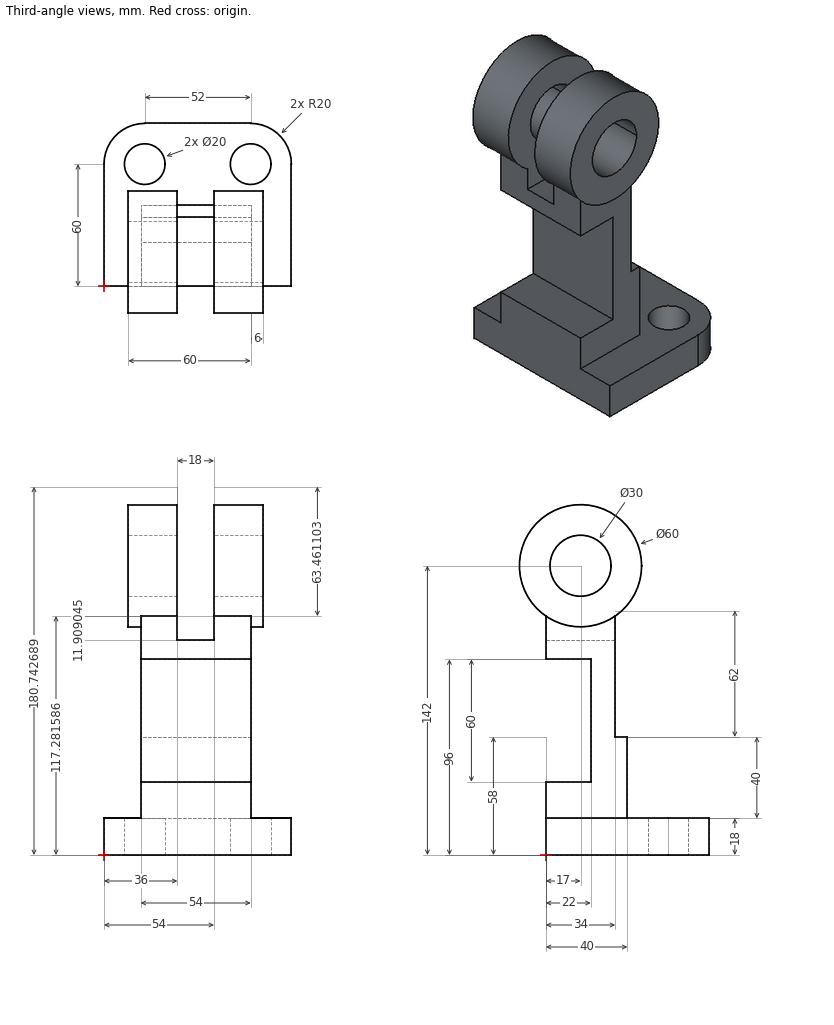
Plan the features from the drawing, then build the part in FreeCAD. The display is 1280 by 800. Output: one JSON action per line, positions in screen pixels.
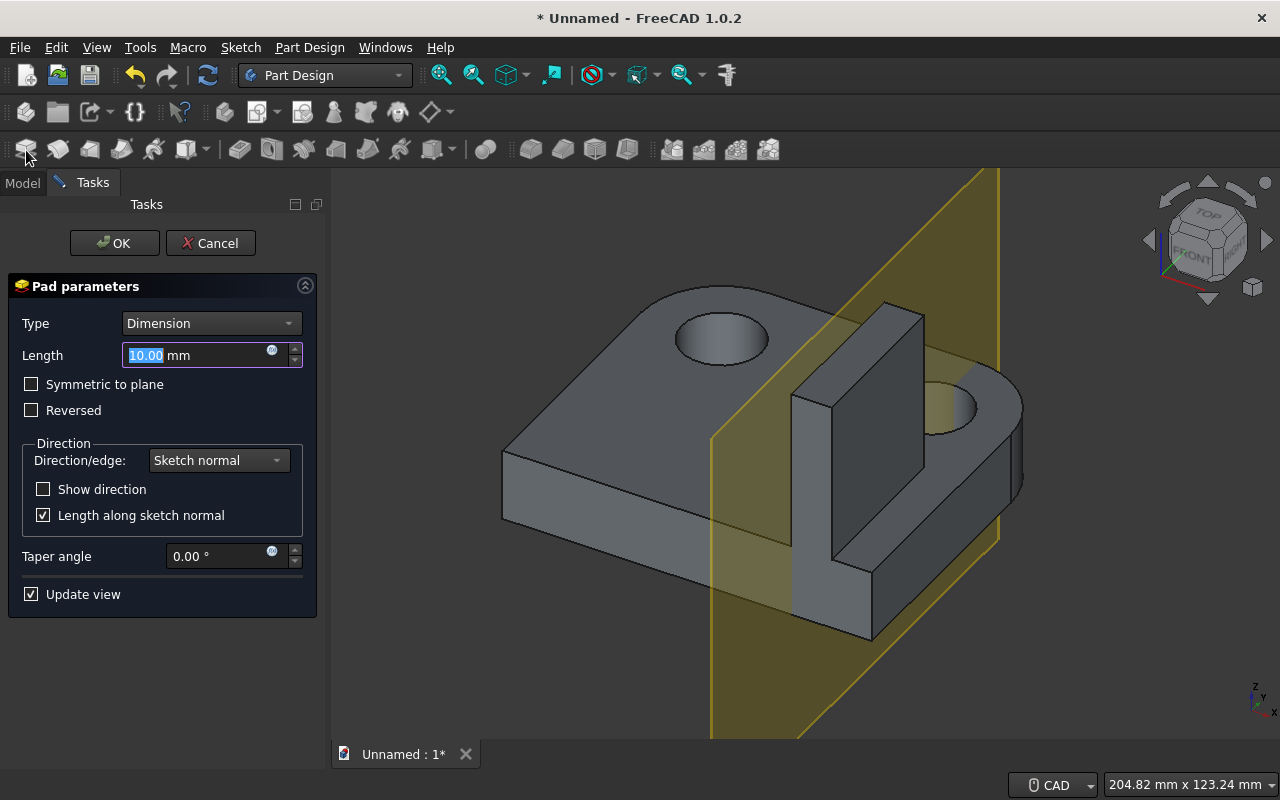
{"action": "type", "text": "54"}
{"action": "key", "text": "Tab"}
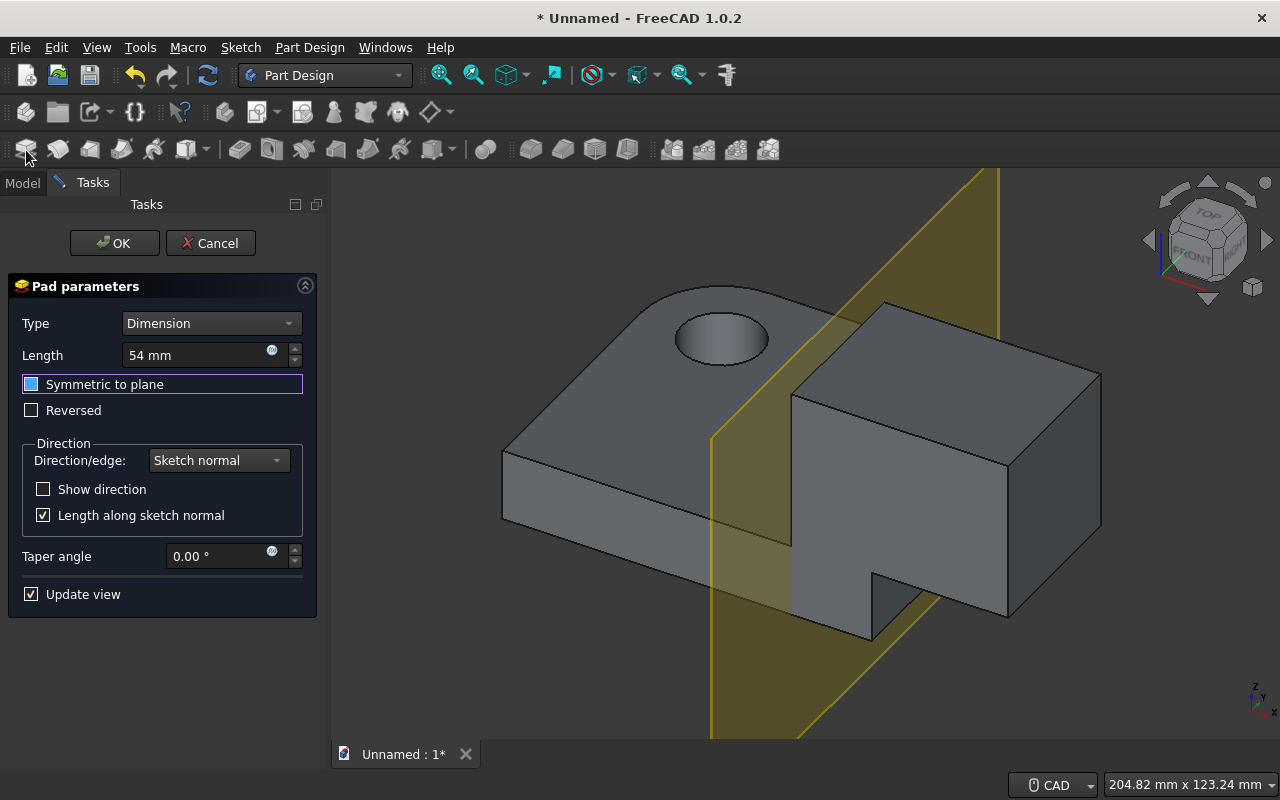
{"action": "left_click", "coordinate": [30, 410]}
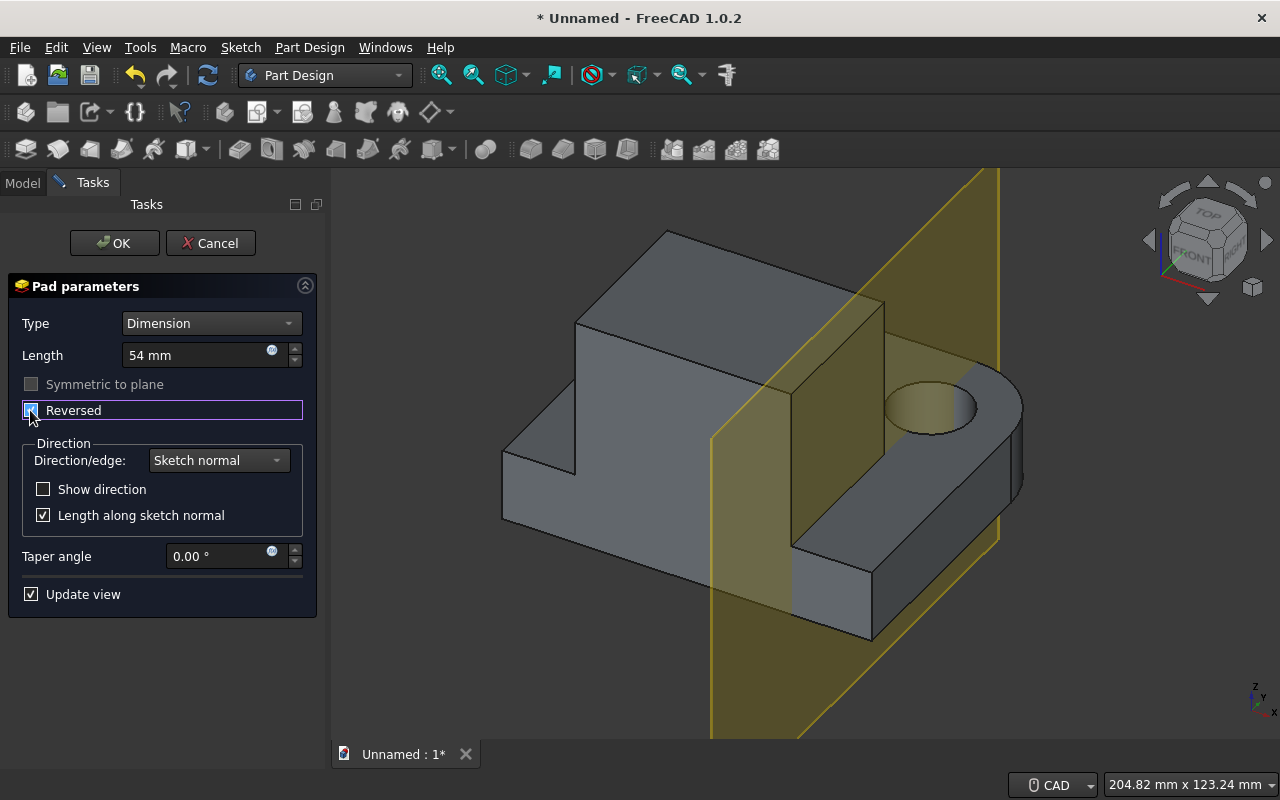
{"action": "left_click", "coordinate": [115, 243]}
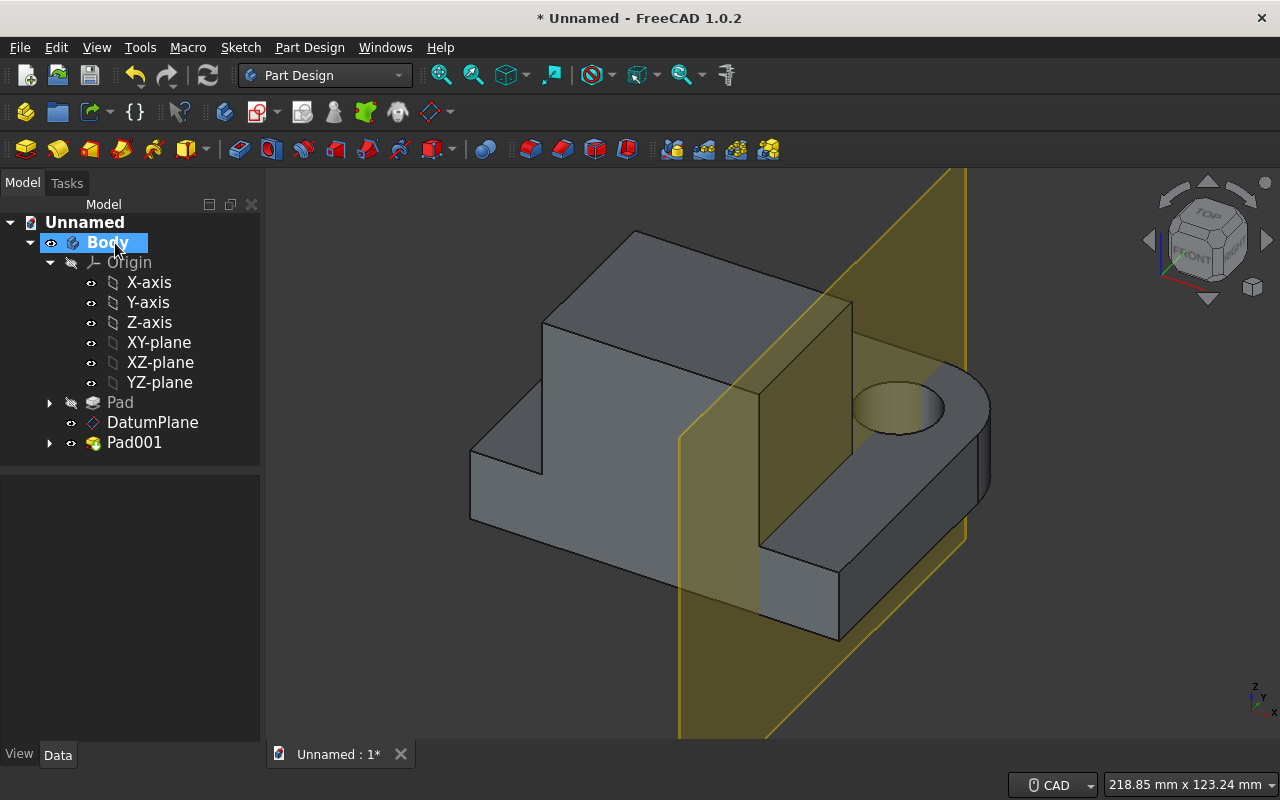
{"action": "left_click", "coordinate": [116, 423]}
{"action": "key", "text": "space"}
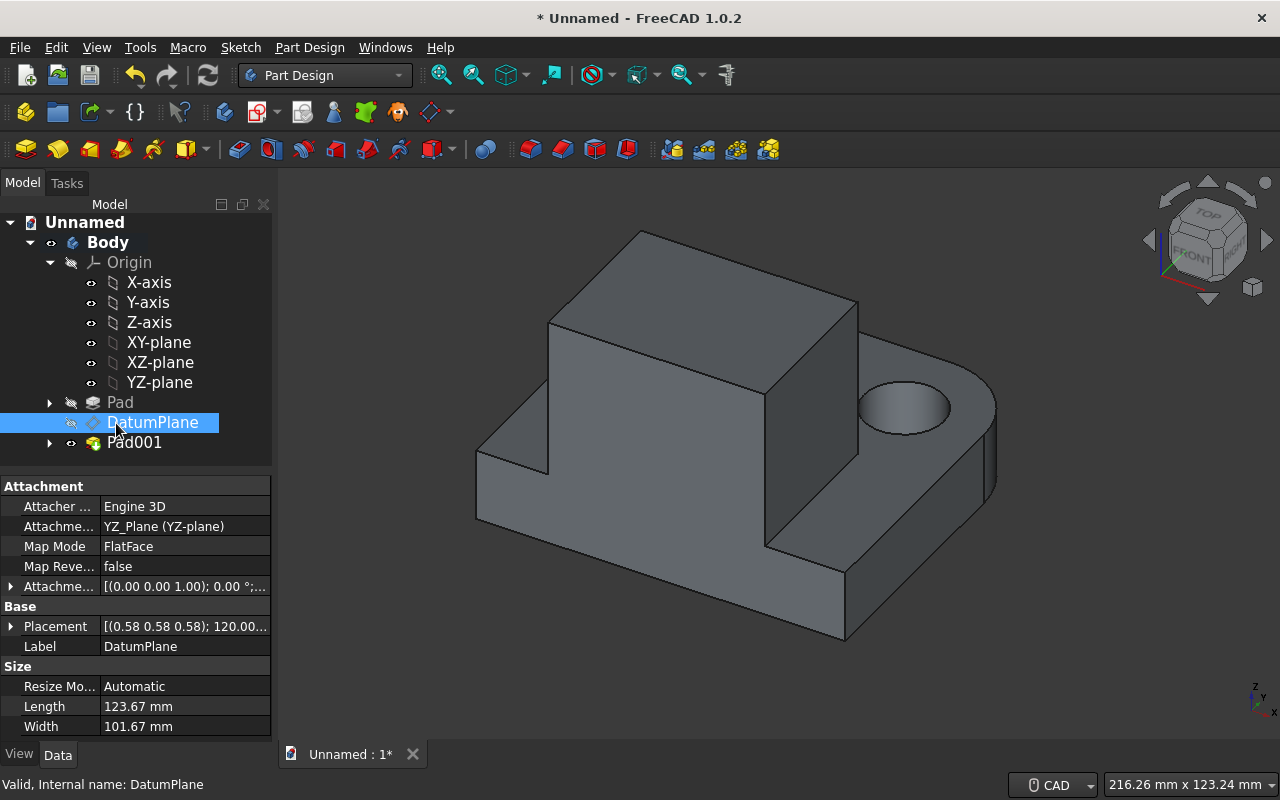
{"action": "left_click", "coordinate": [442, 76]}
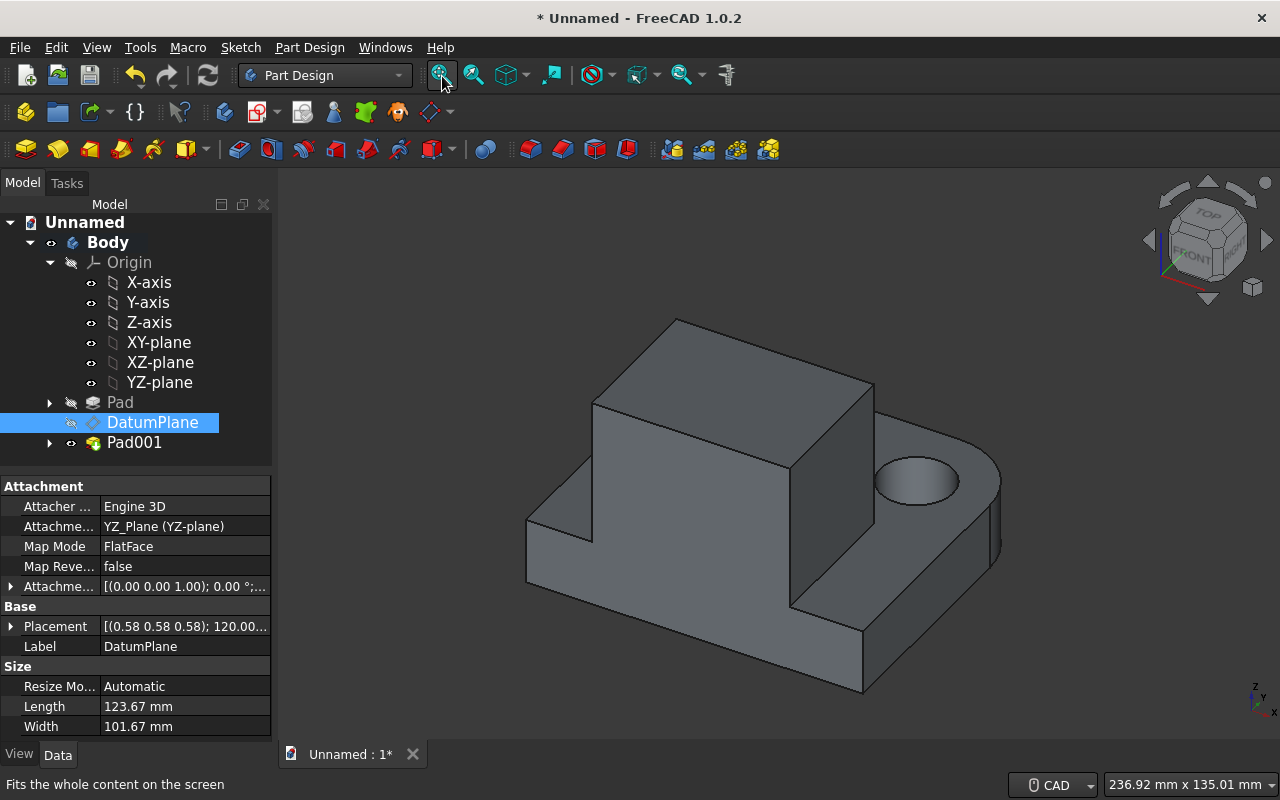
{"action": "left_click", "coordinate": [832, 495]}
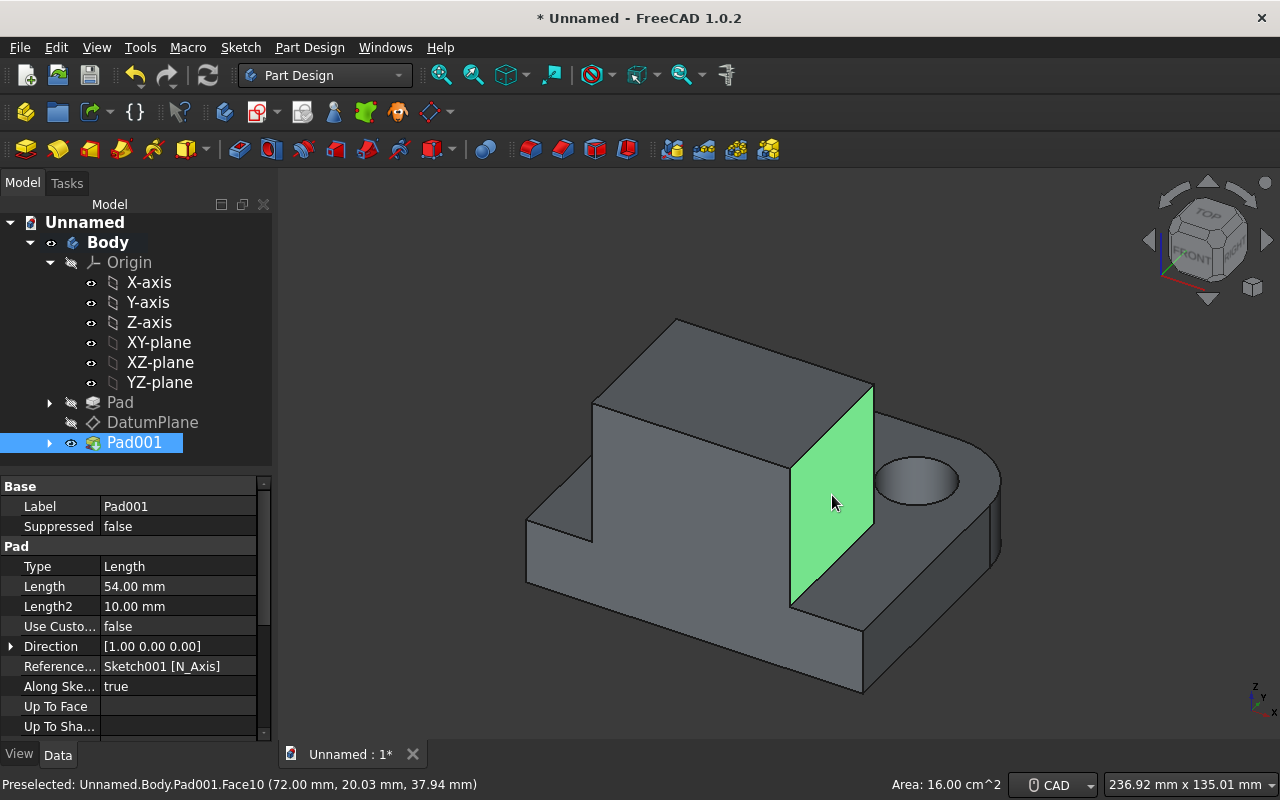
{"action": "left_click", "coordinate": [258, 112]}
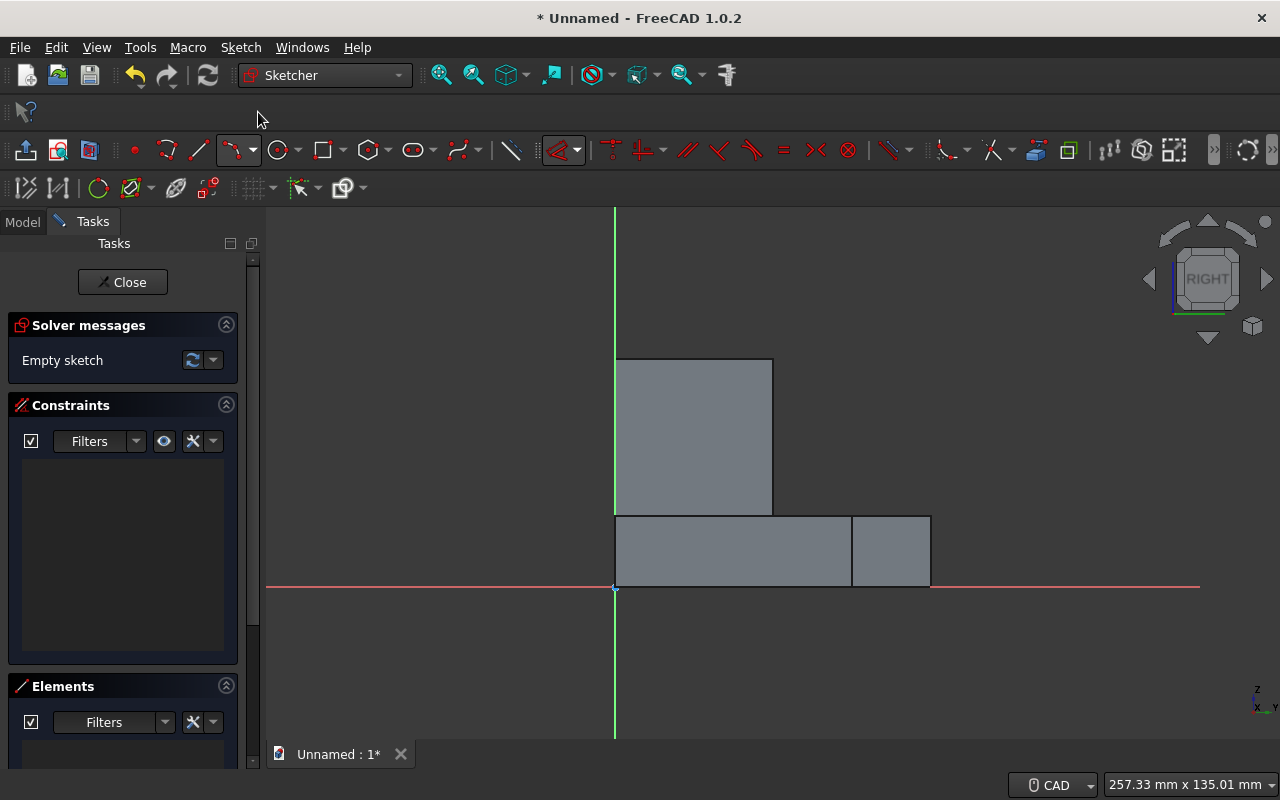
{"action": "left_click", "coordinate": [90, 150]}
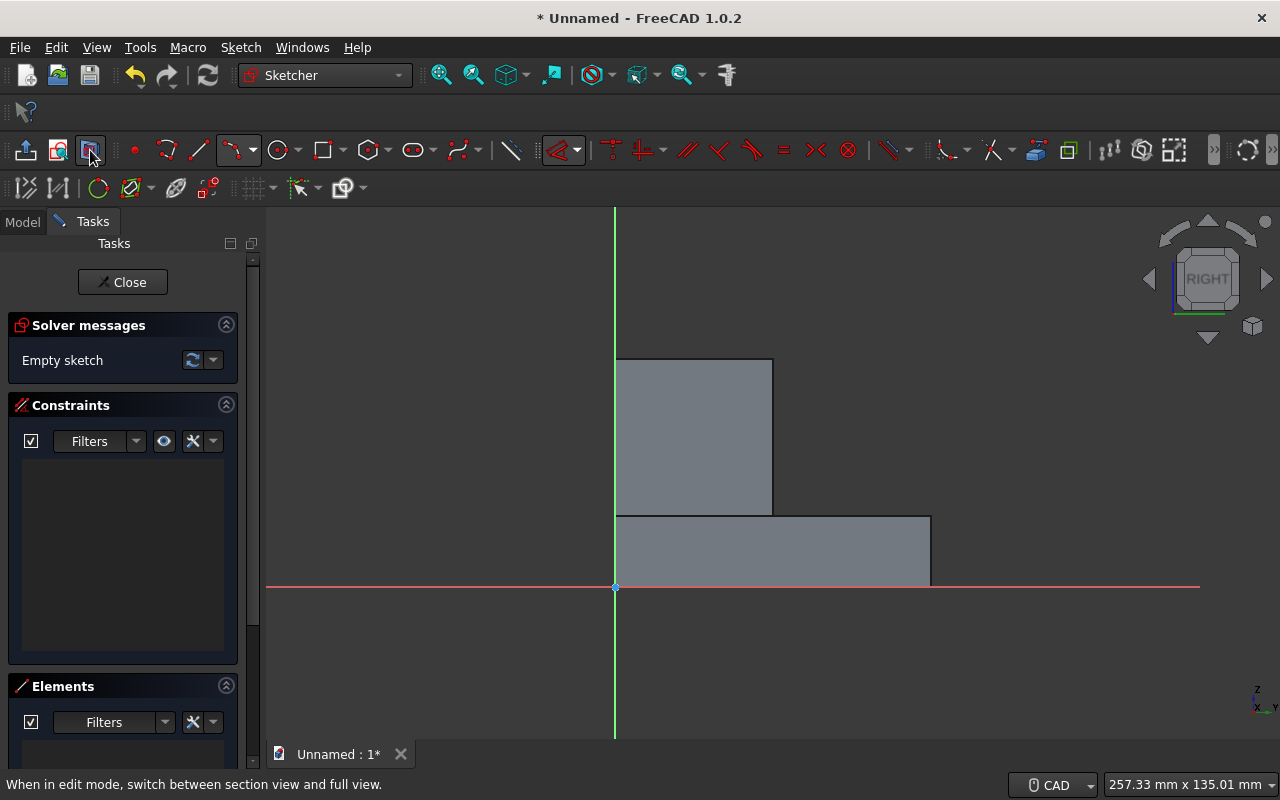
{"action": "scroll", "coordinate": [749, 711], "scroll_direction": "down", "scroll_amount": 2}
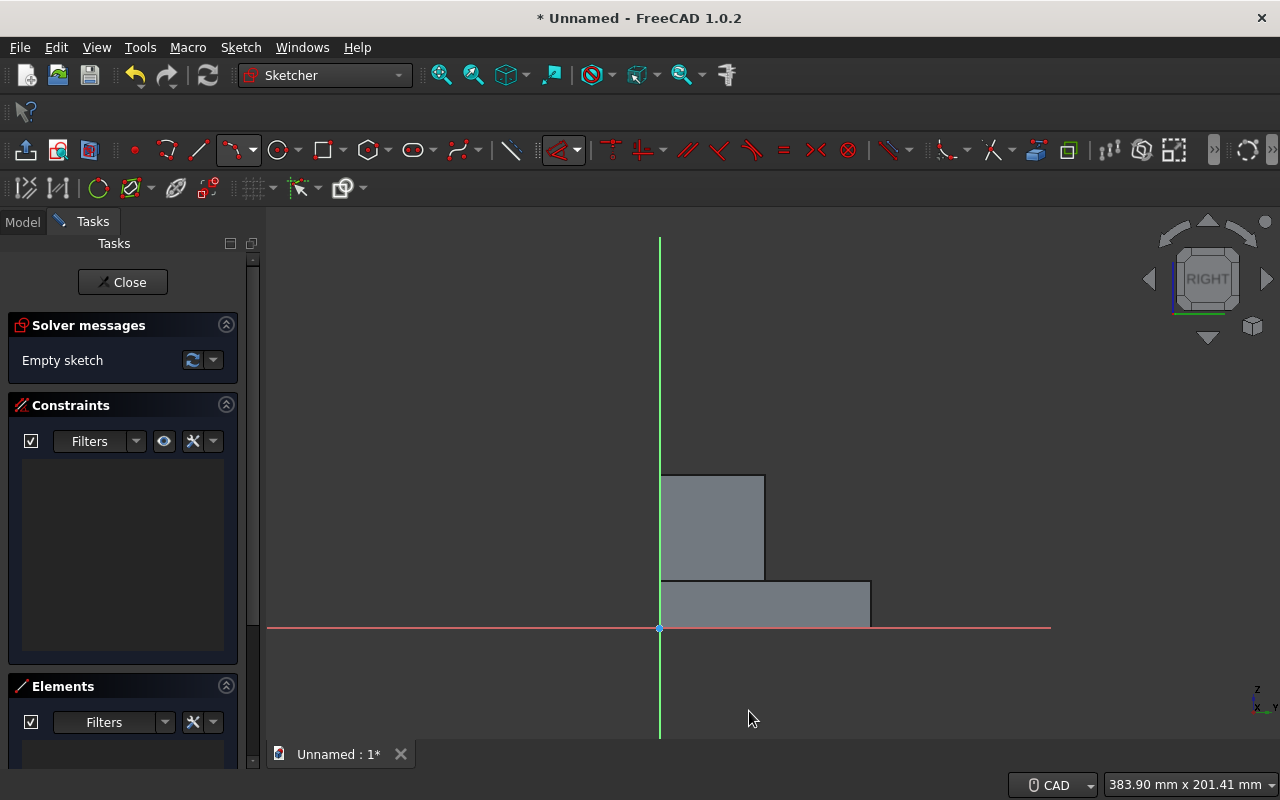
{"action": "left_click", "coordinate": [324, 150]}